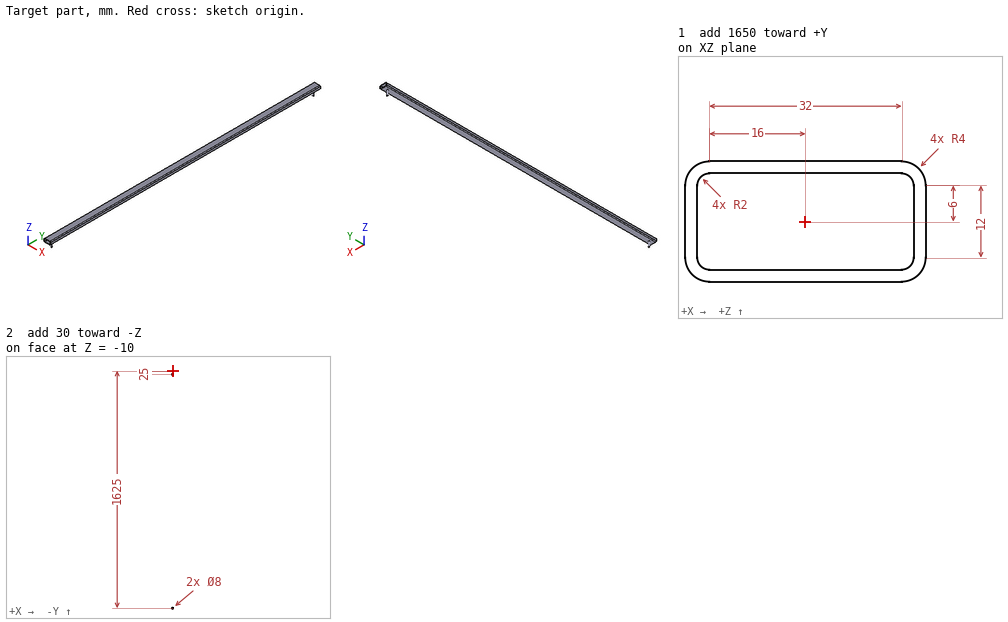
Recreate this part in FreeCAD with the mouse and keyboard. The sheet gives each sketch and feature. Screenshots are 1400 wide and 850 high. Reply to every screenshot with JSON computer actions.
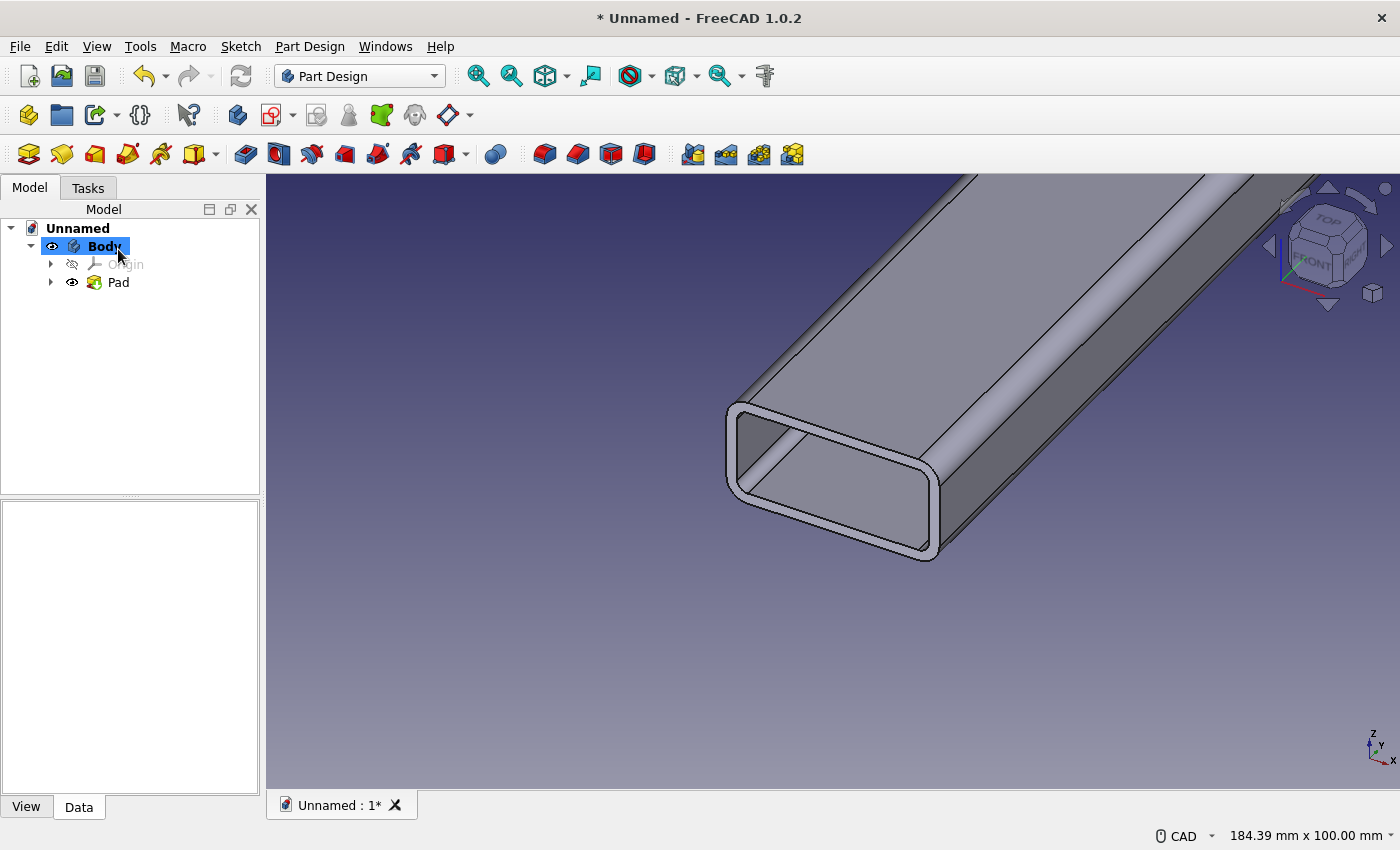
{"action": "left_click", "coordinate": [479, 76]}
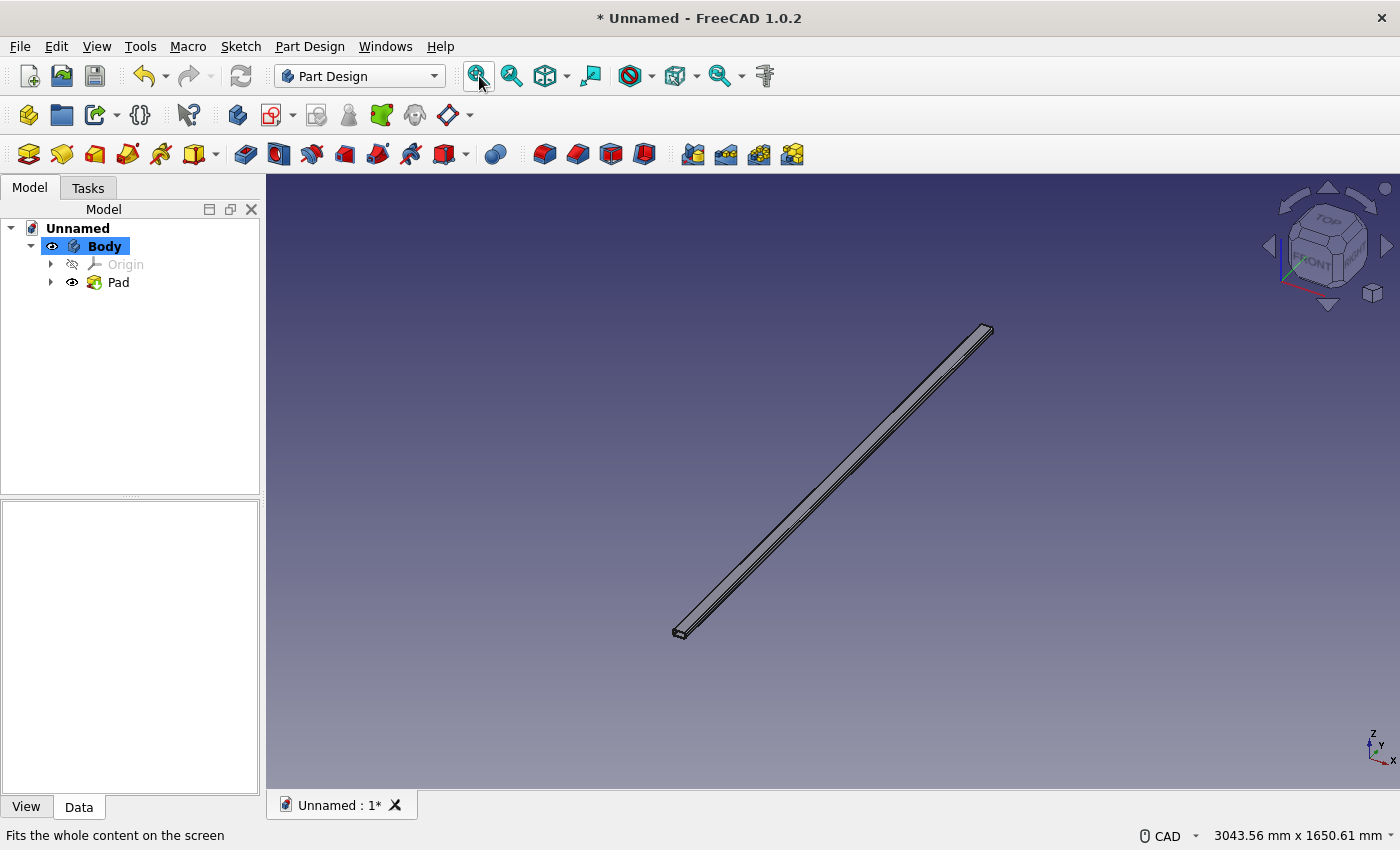
{"action": "key", "text": "5"}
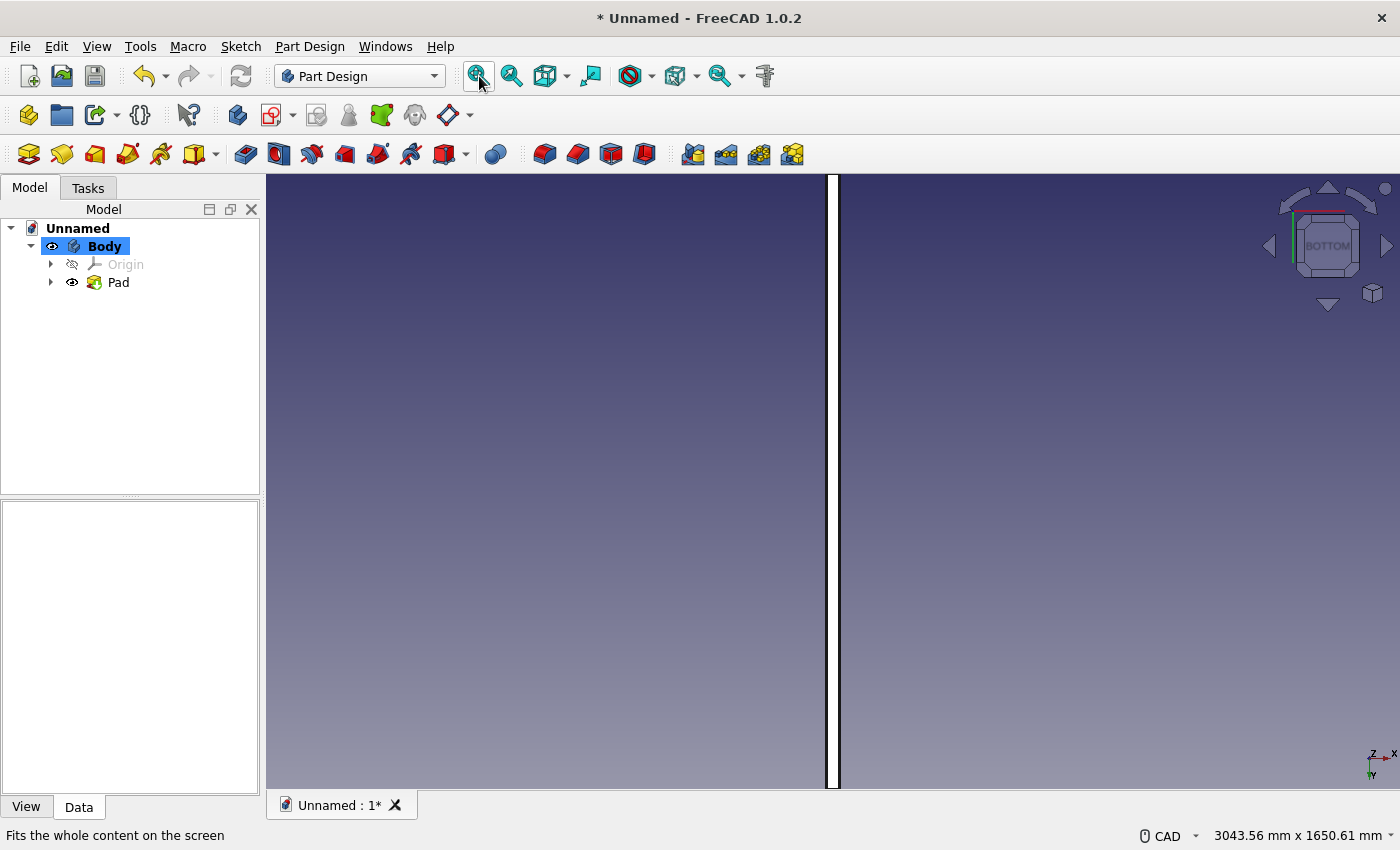
{"action": "left_click", "coordinate": [479, 76]}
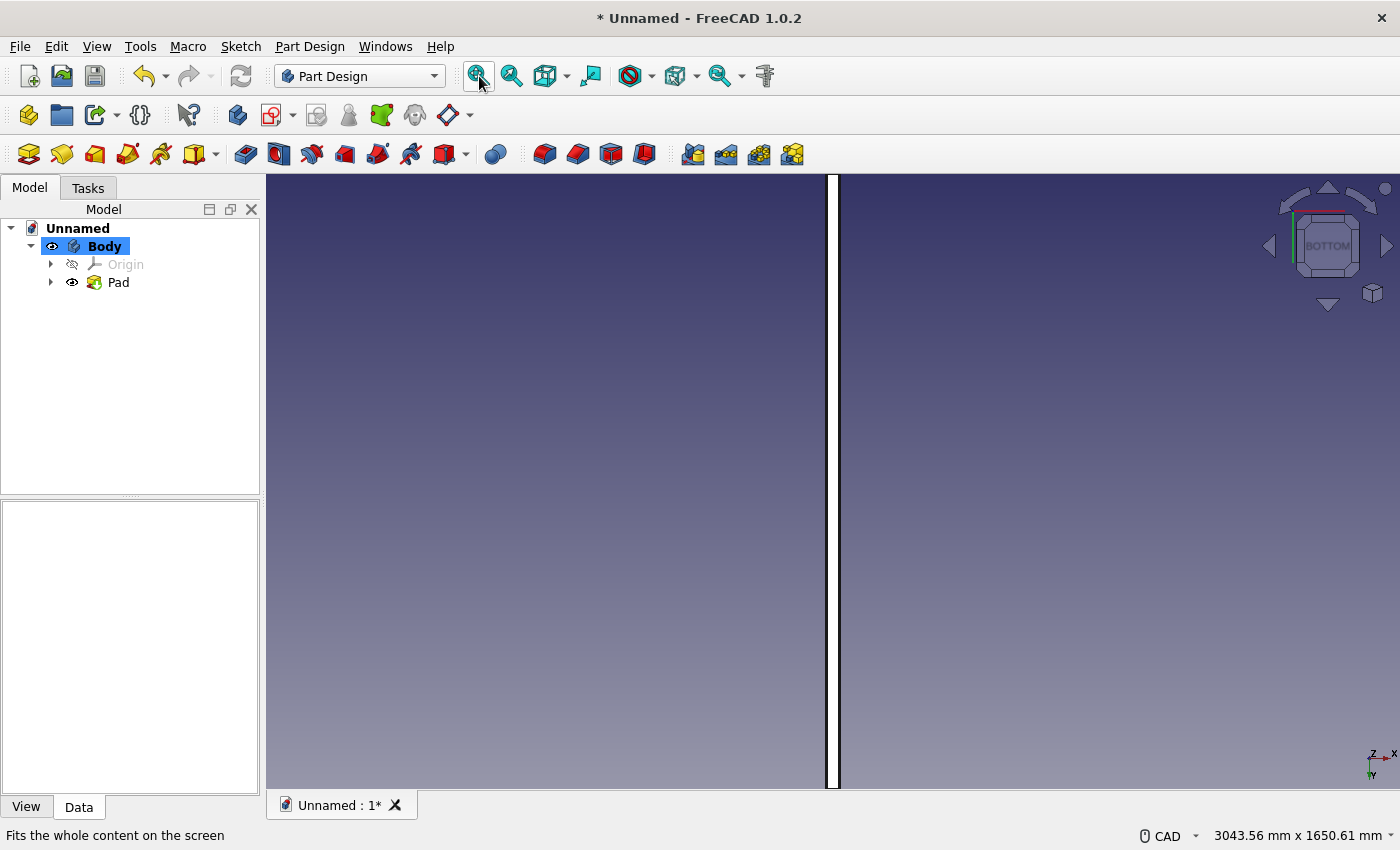
{"action": "scroll", "coordinate": [833, 744], "scroll_direction": "up", "scroll_amount": 4}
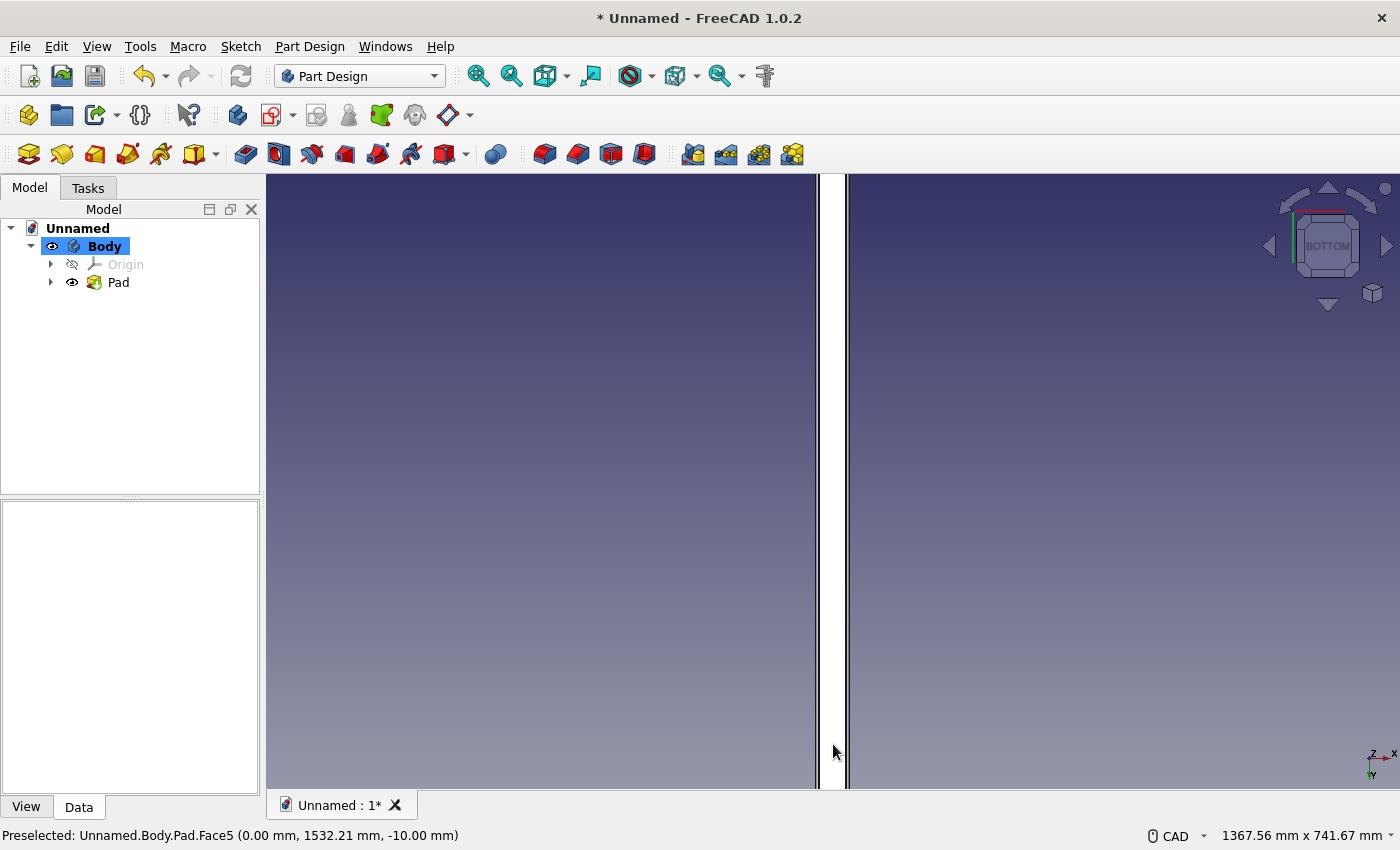
{"action": "left_click", "coordinate": [832, 744]}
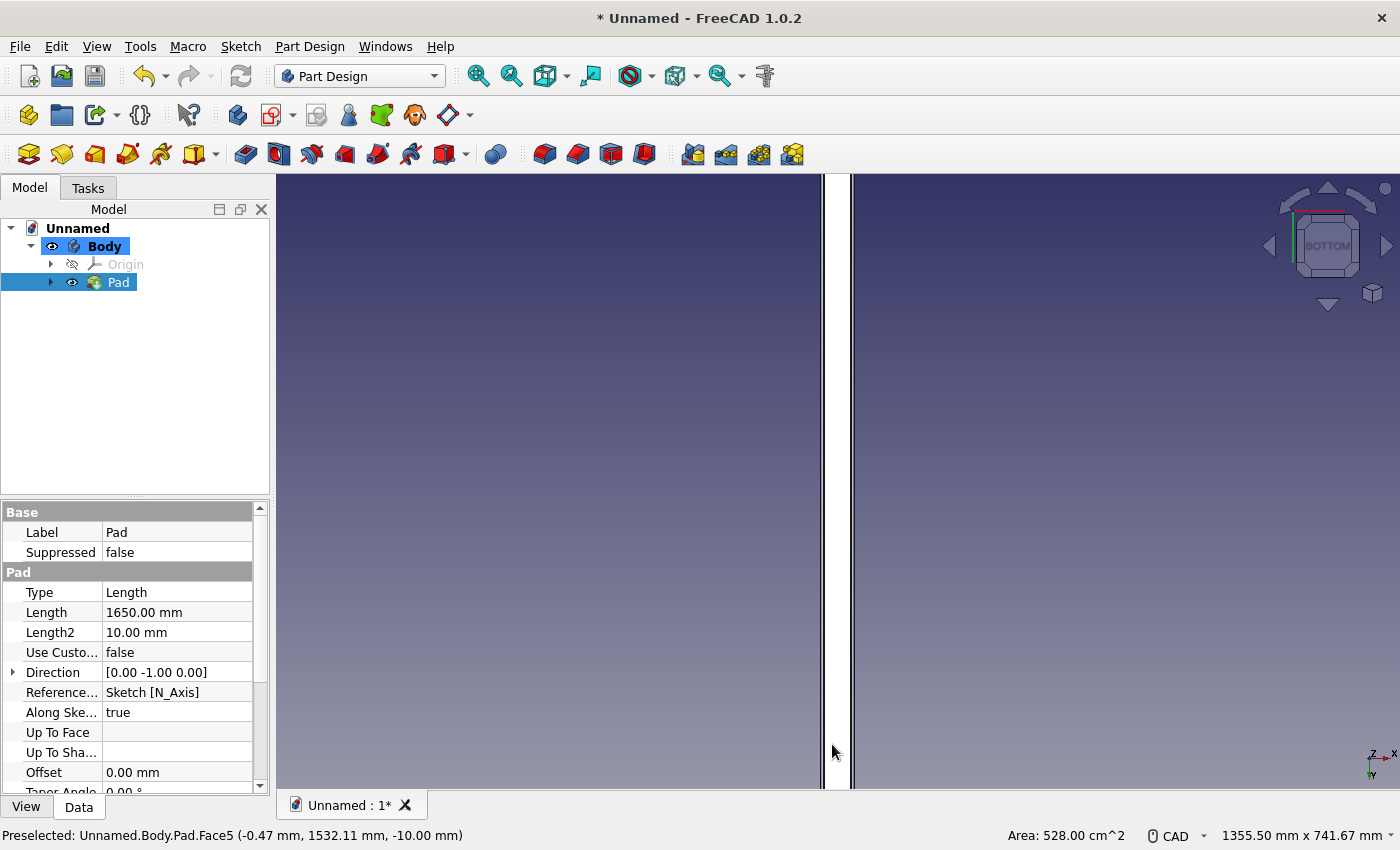
{"action": "left_click", "coordinate": [270, 116]}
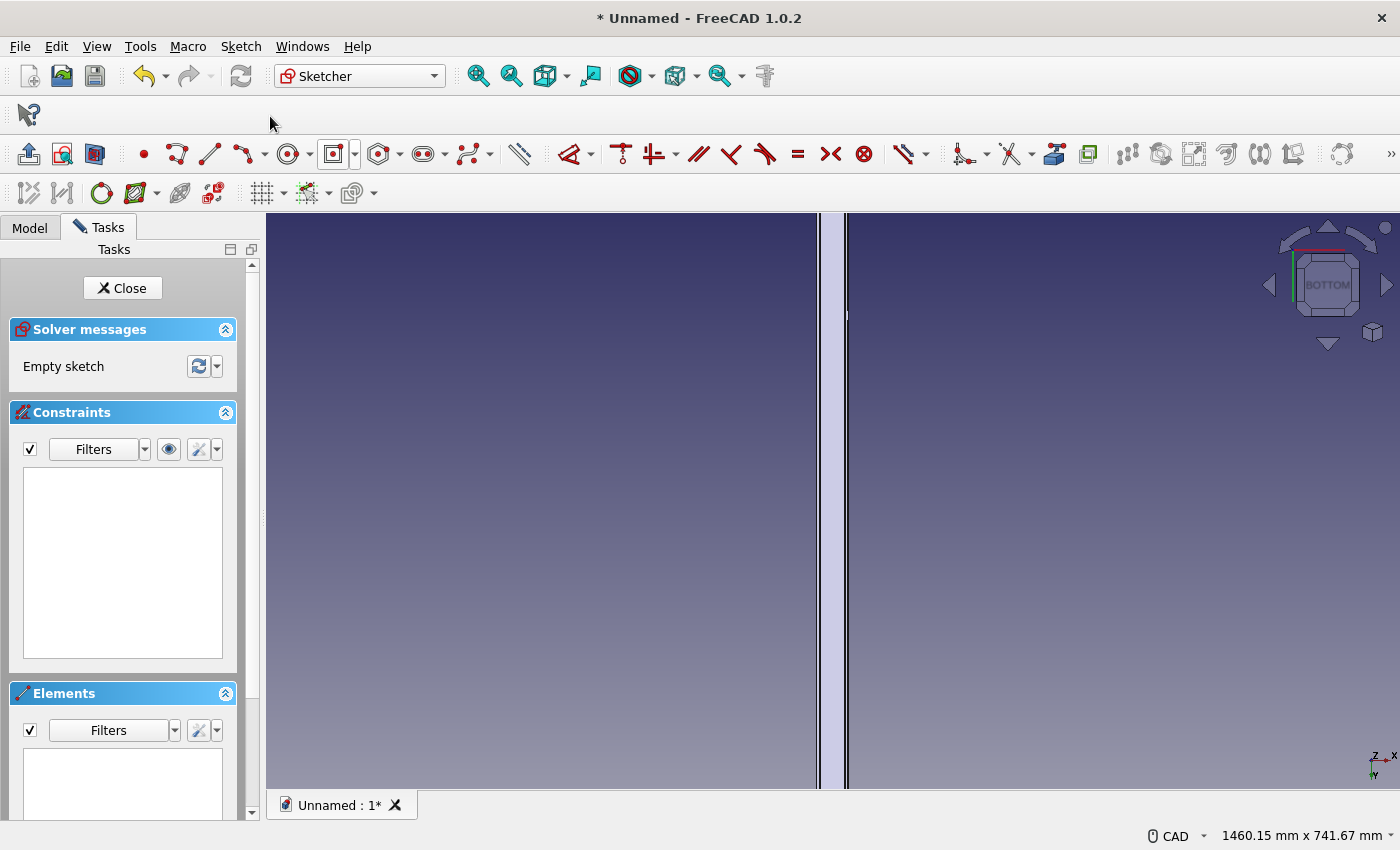
{"action": "scroll", "coordinate": [735, 635], "scroll_direction": "down", "scroll_amount": 6}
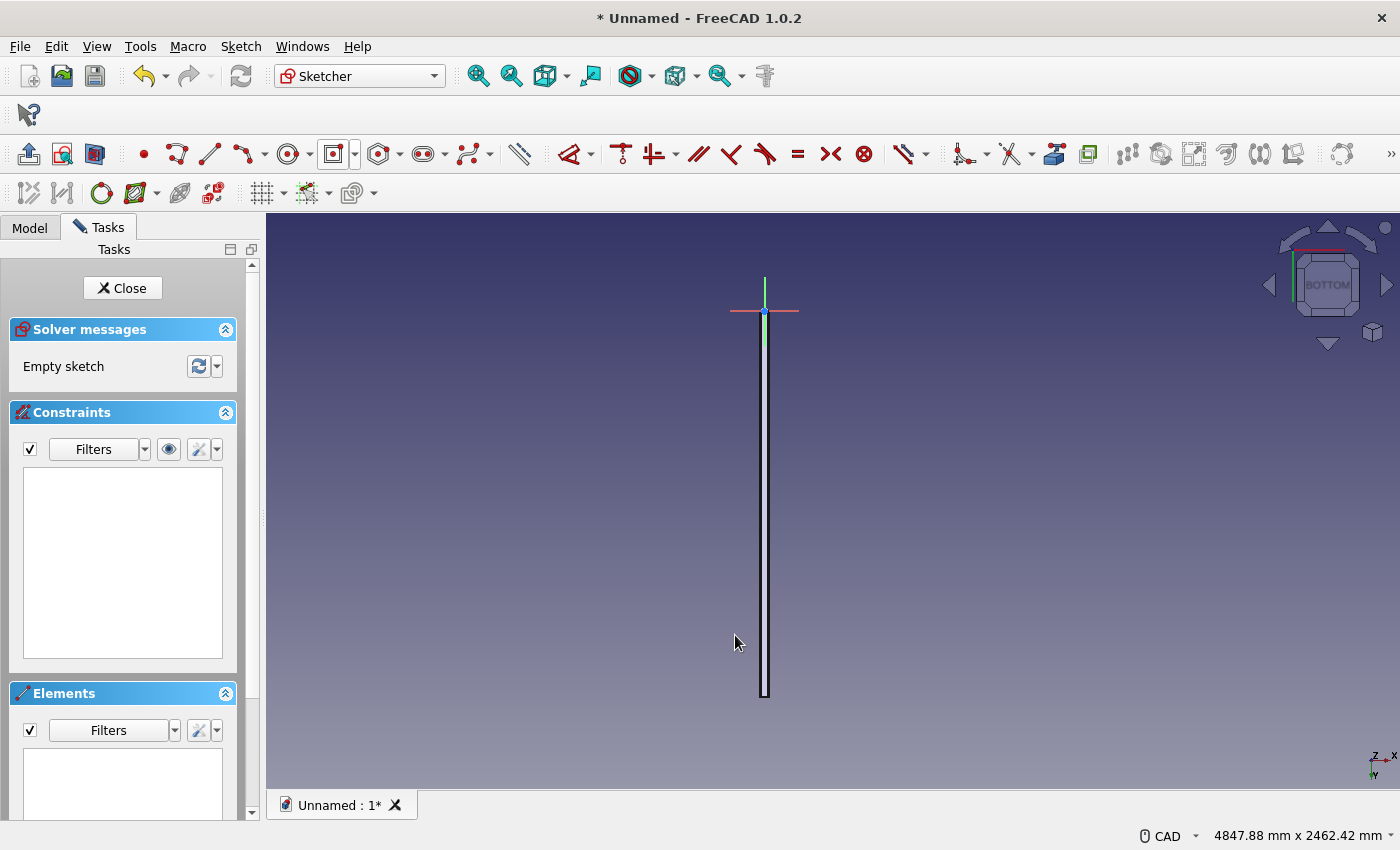
{"action": "left_click", "coordinate": [288, 154]}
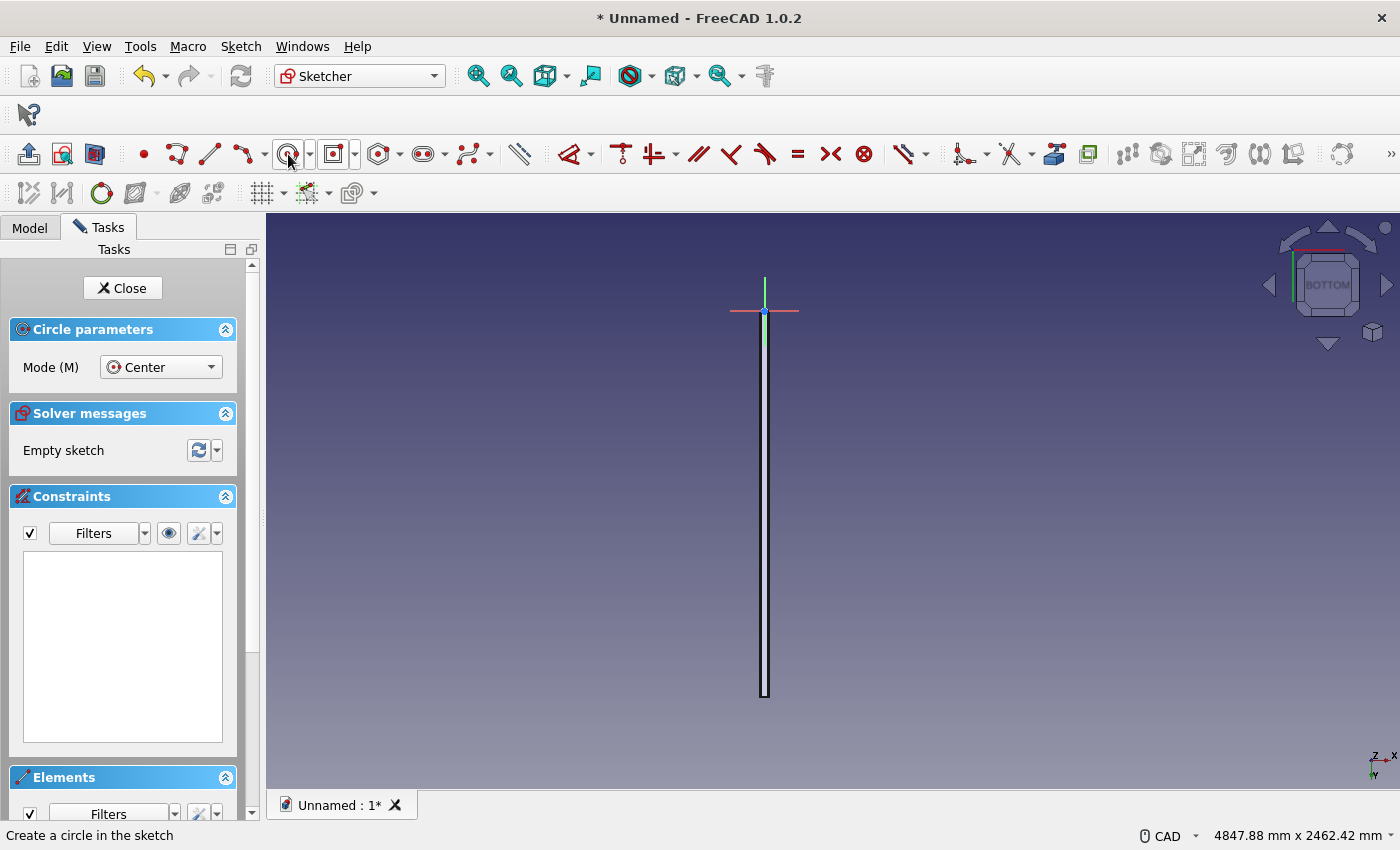
{"action": "scroll", "coordinate": [765, 691], "scroll_direction": "up", "scroll_amount": 16}